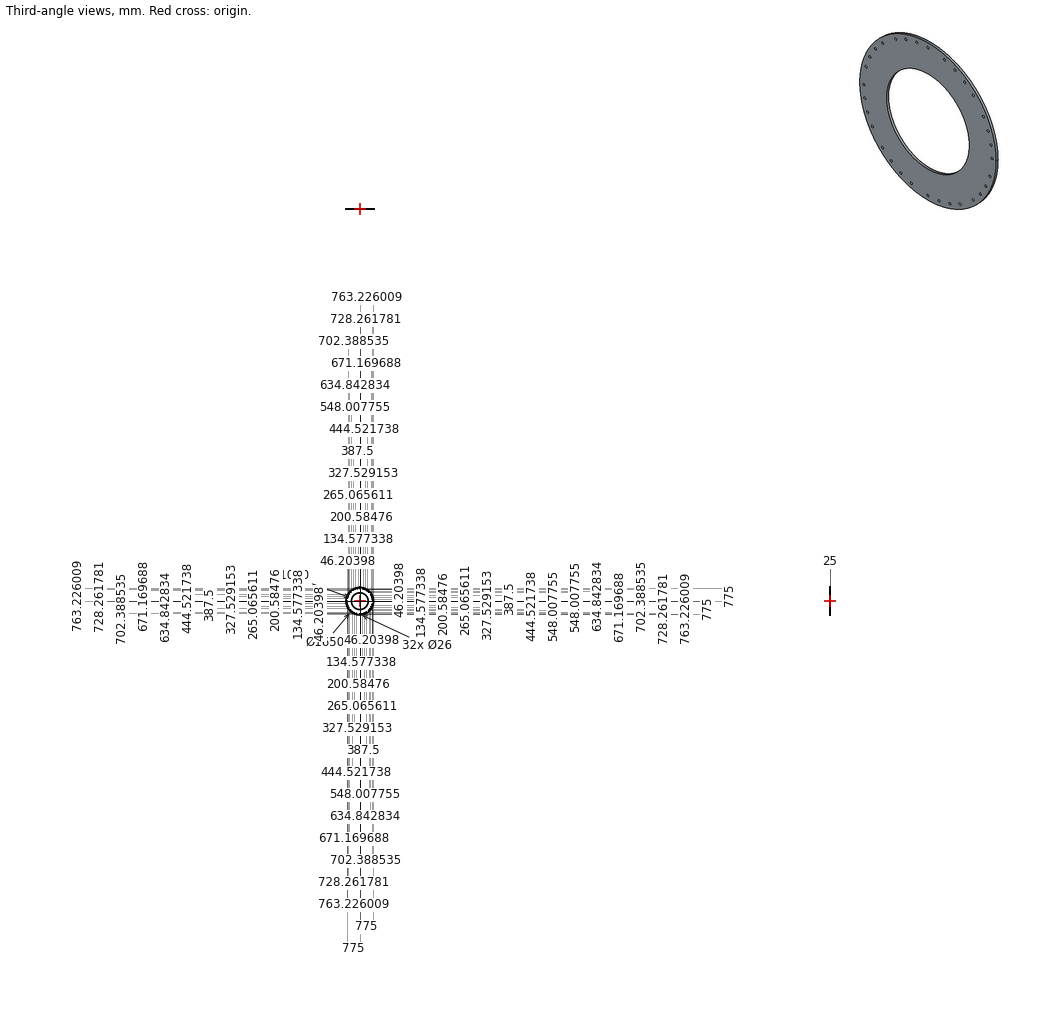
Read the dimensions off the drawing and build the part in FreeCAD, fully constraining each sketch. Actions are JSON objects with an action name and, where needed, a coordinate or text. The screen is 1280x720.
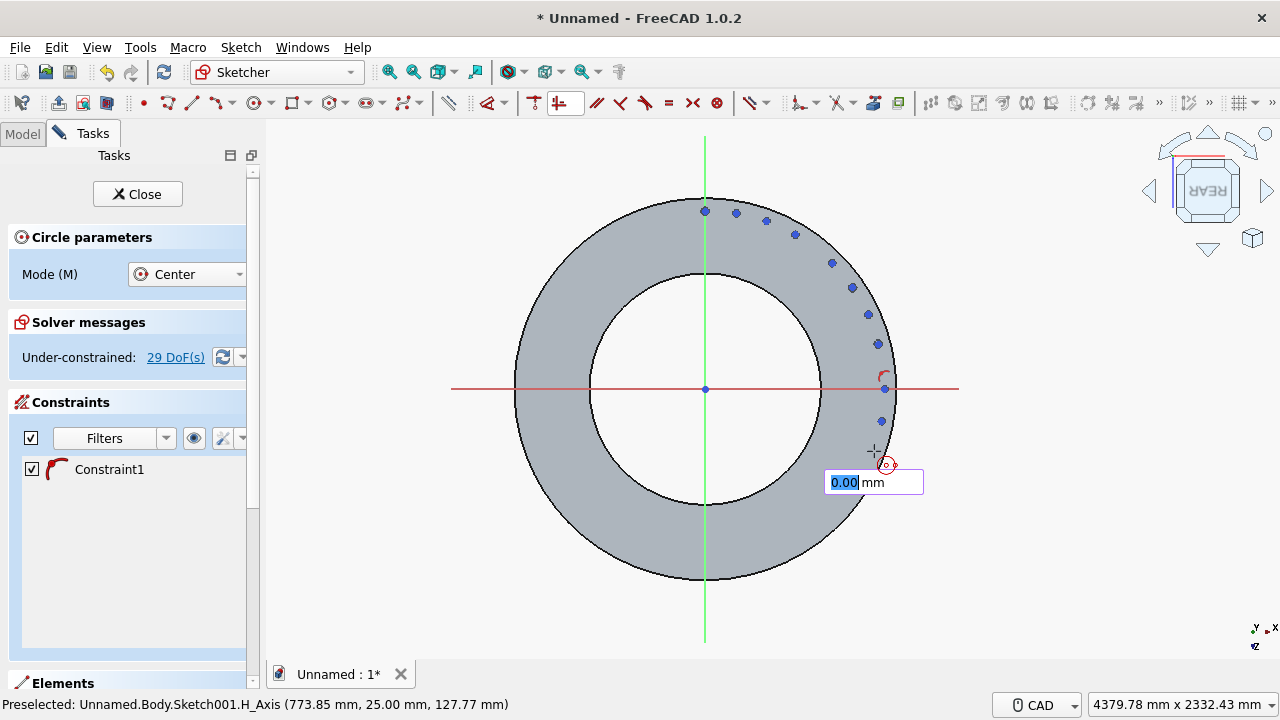
{"action": "scroll", "coordinate": [876, 448], "scroll_direction": "up", "scroll_amount": 9}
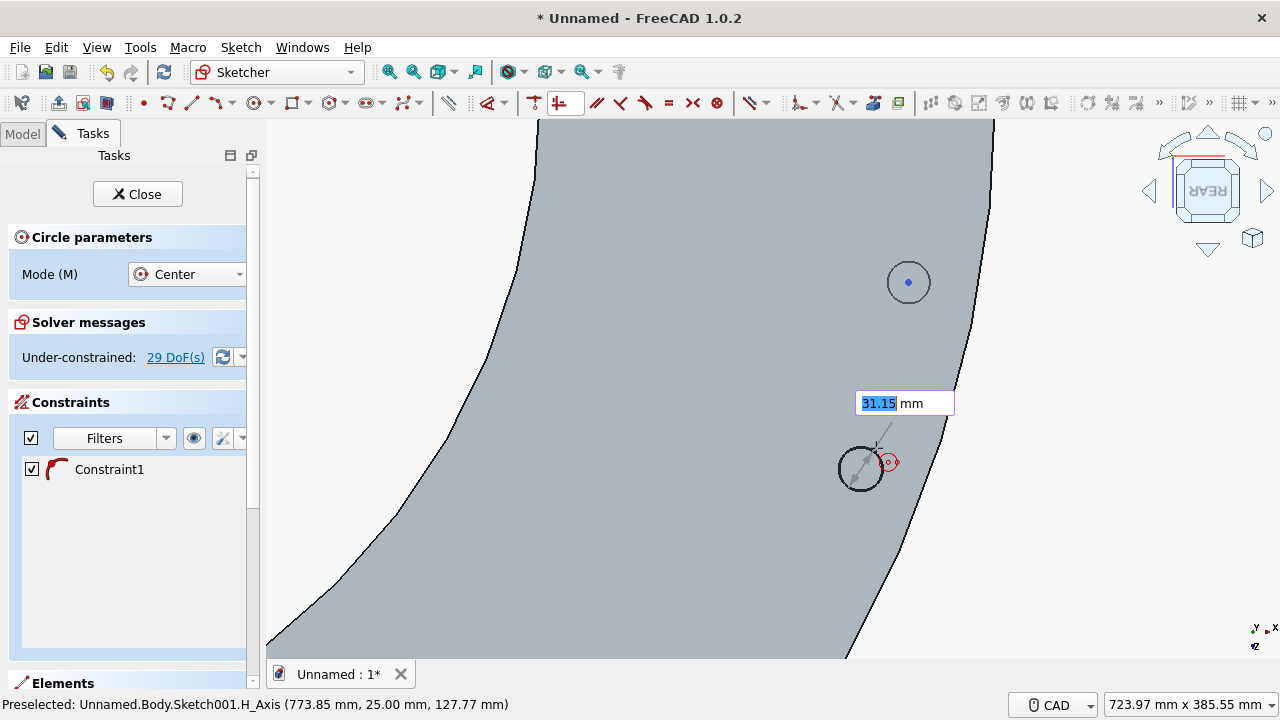
{"action": "left_click", "coordinate": [873, 448]}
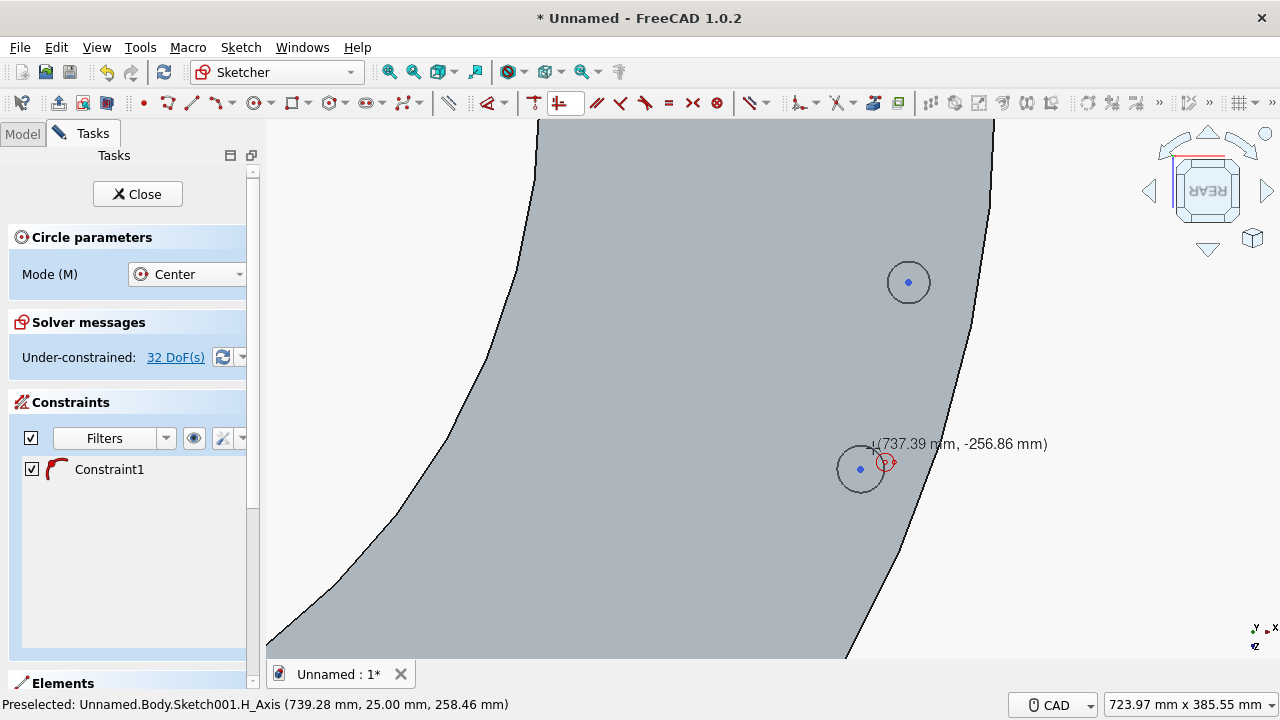
{"action": "scroll", "coordinate": [876, 448], "scroll_direction": "down", "scroll_amount": 9}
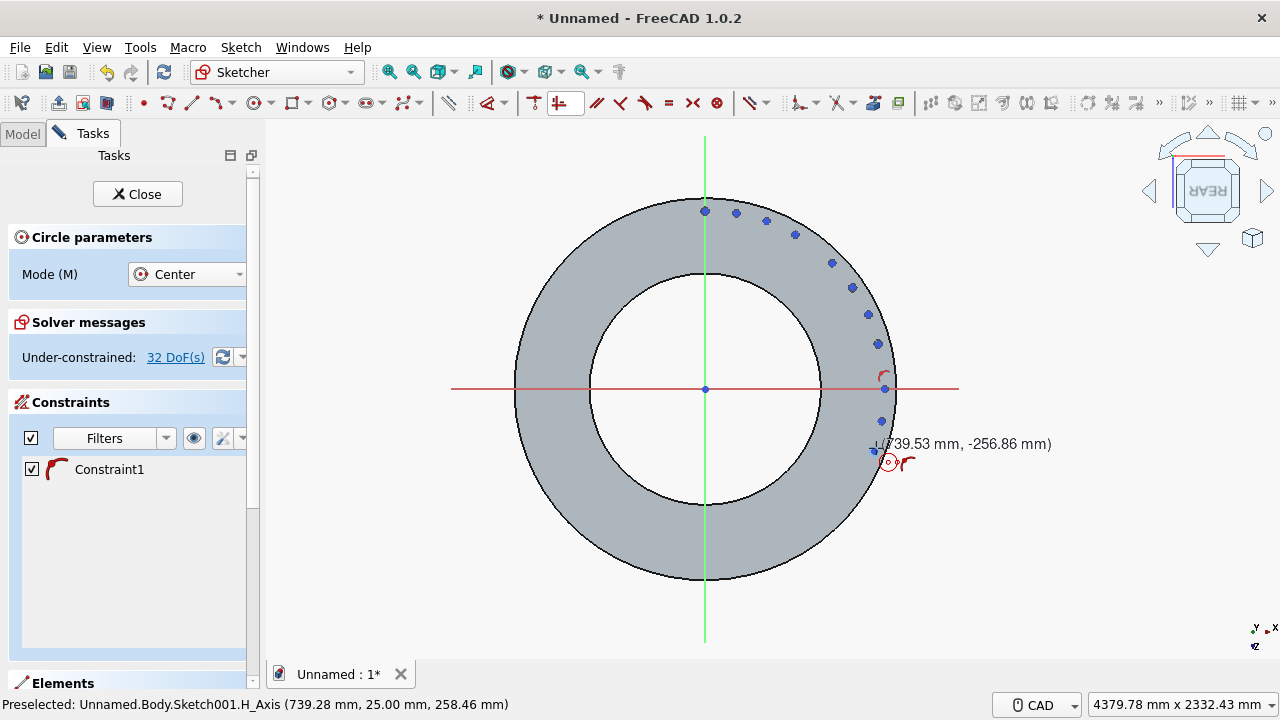
{"action": "scroll", "coordinate": [861, 479], "scroll_direction": "up", "scroll_amount": 11}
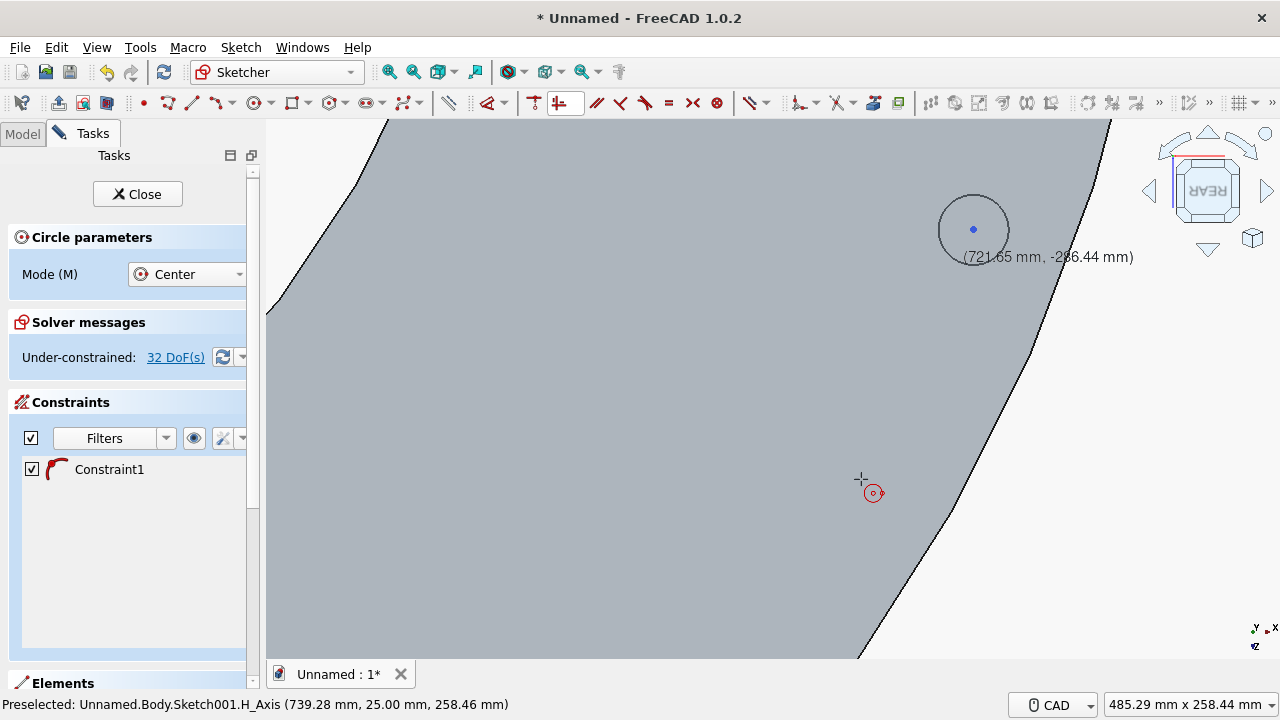
{"action": "scroll", "coordinate": [861, 479], "scroll_direction": "down", "scroll_amount": 11}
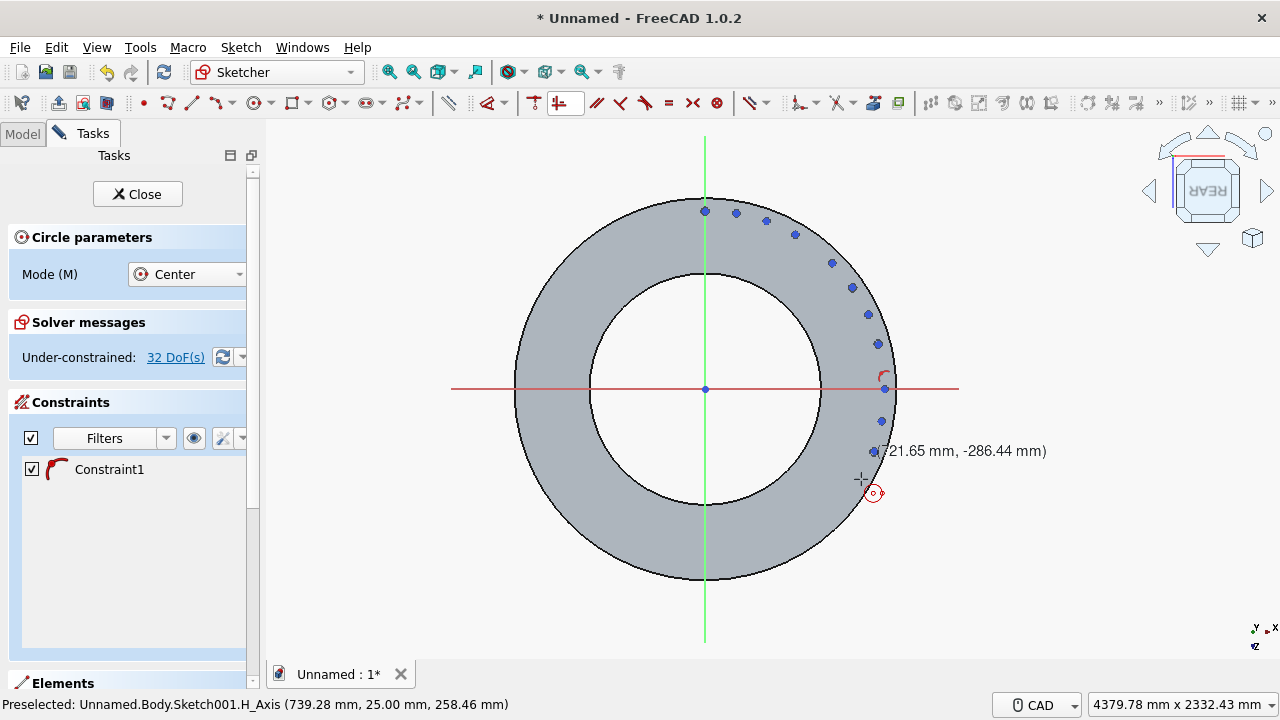
{"action": "left_click", "coordinate": [861, 479]}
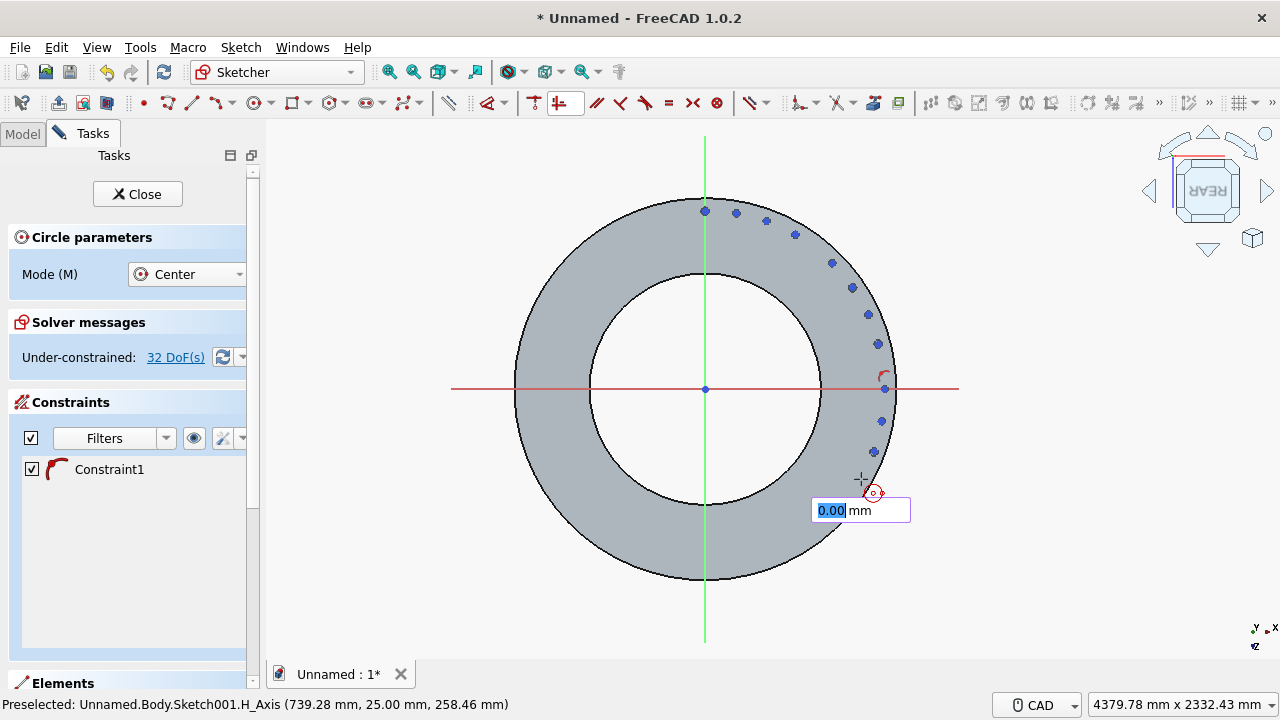
{"action": "scroll", "coordinate": [863, 477], "scroll_direction": "up", "scroll_amount": 9}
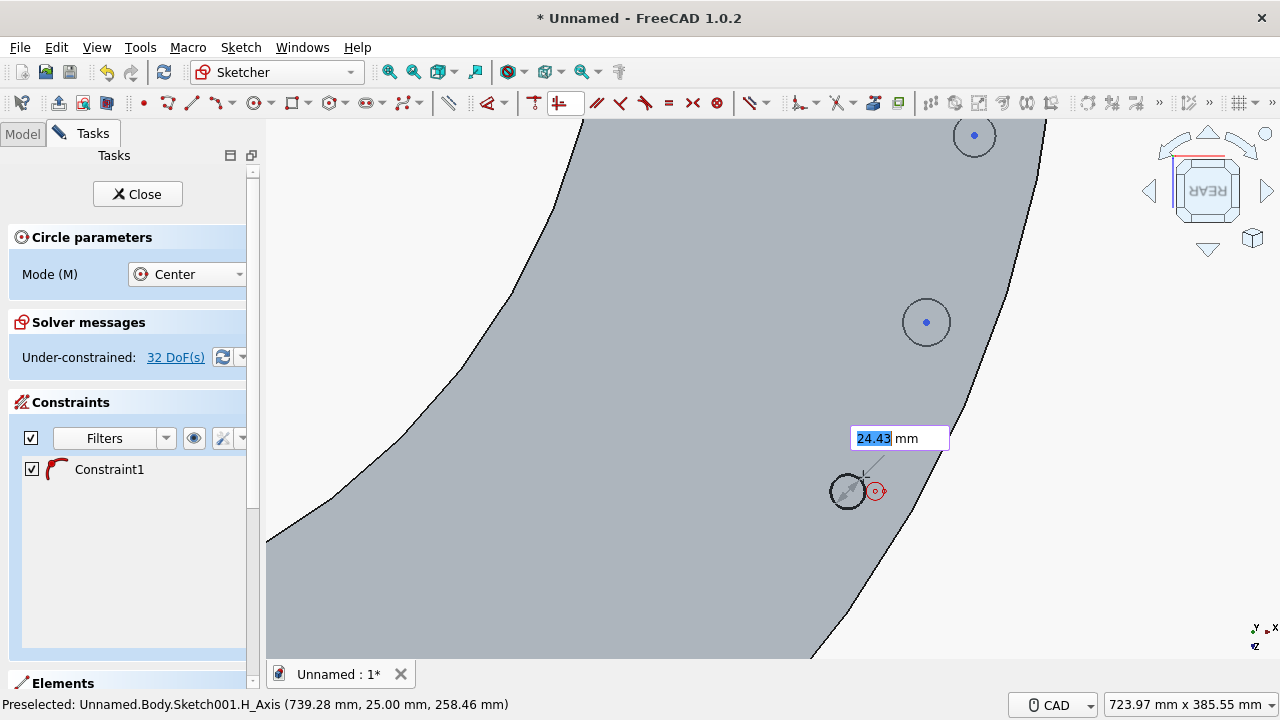
{"action": "left_click", "coordinate": [859, 472]}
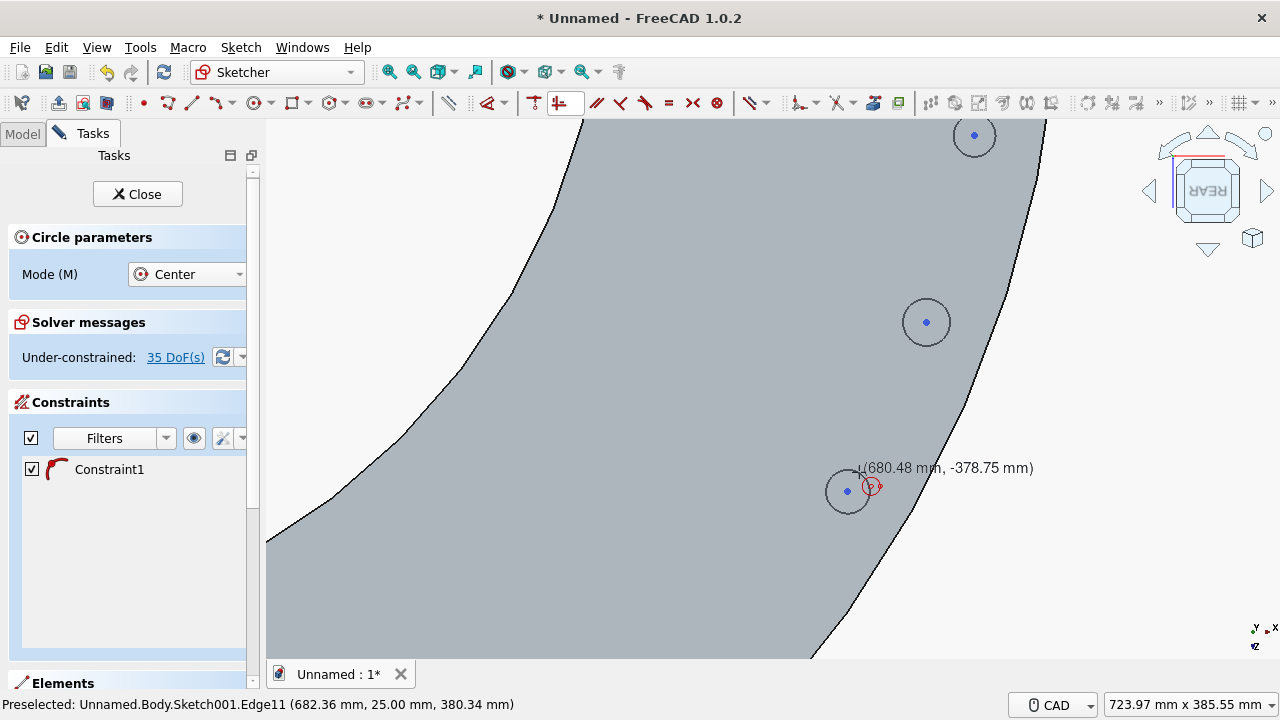
{"action": "scroll", "coordinate": [863, 477], "scroll_direction": "down", "scroll_amount": 9}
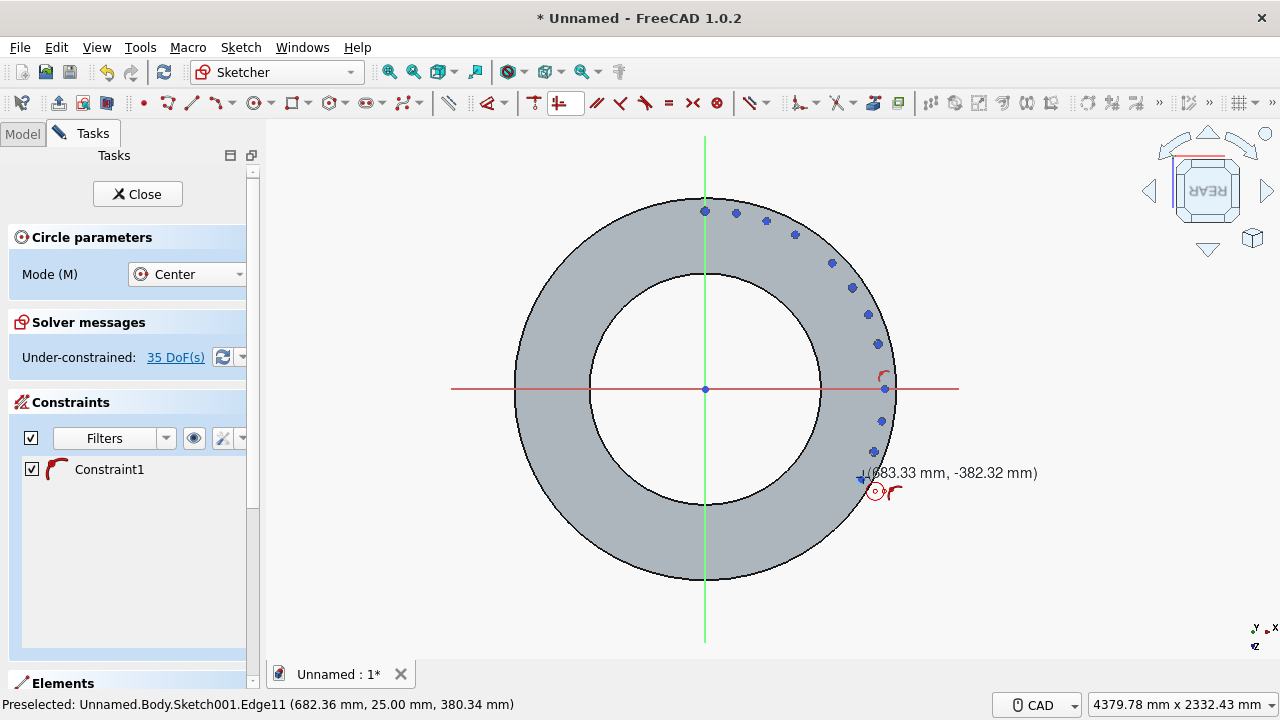
{"action": "scroll", "coordinate": [832, 516], "scroll_direction": "up", "scroll_amount": 11}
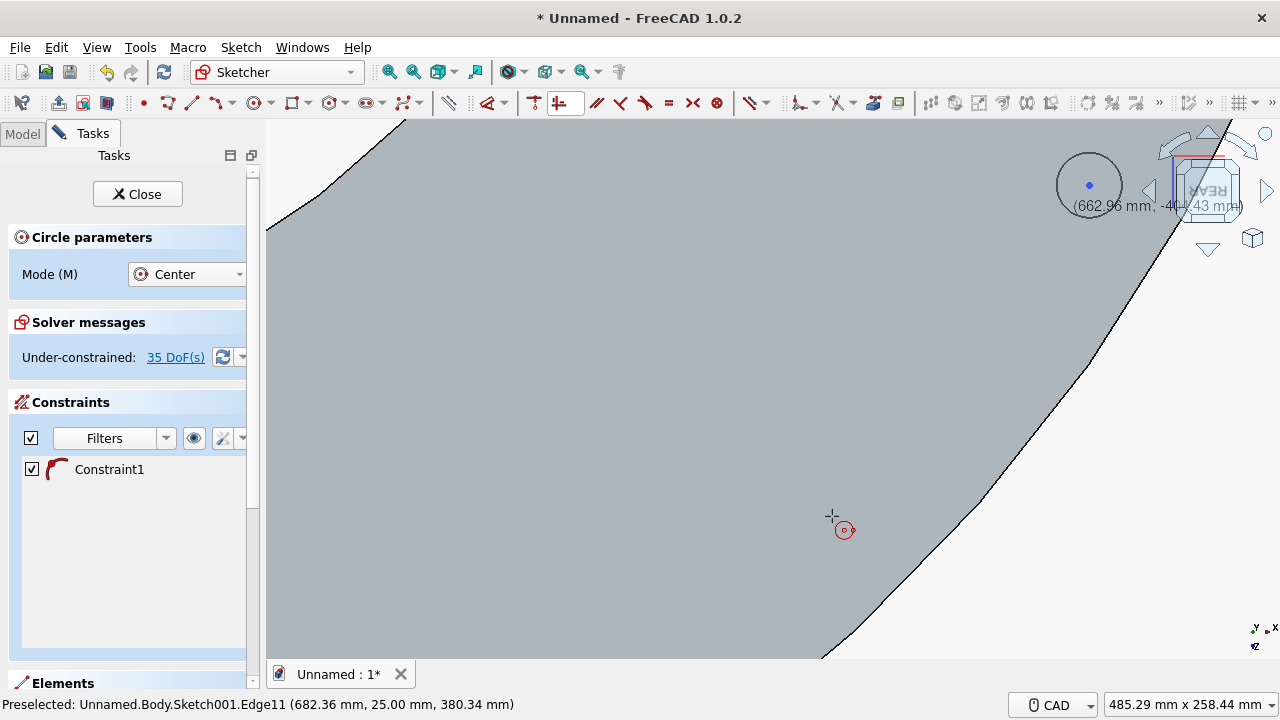
{"action": "scroll", "coordinate": [832, 517], "scroll_direction": "down", "scroll_amount": 11}